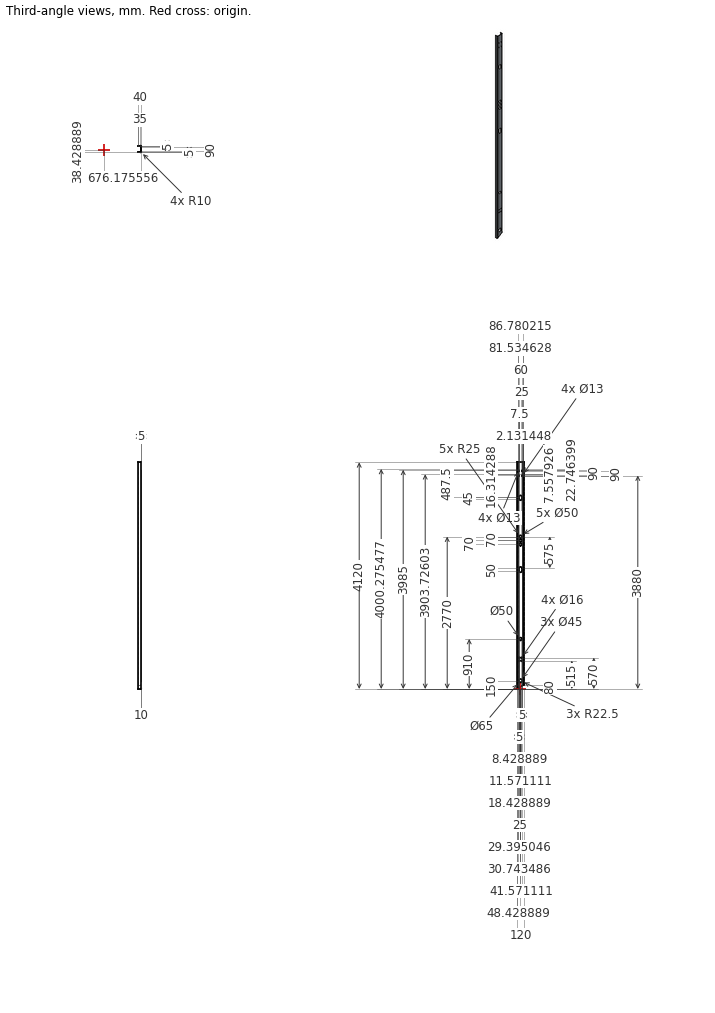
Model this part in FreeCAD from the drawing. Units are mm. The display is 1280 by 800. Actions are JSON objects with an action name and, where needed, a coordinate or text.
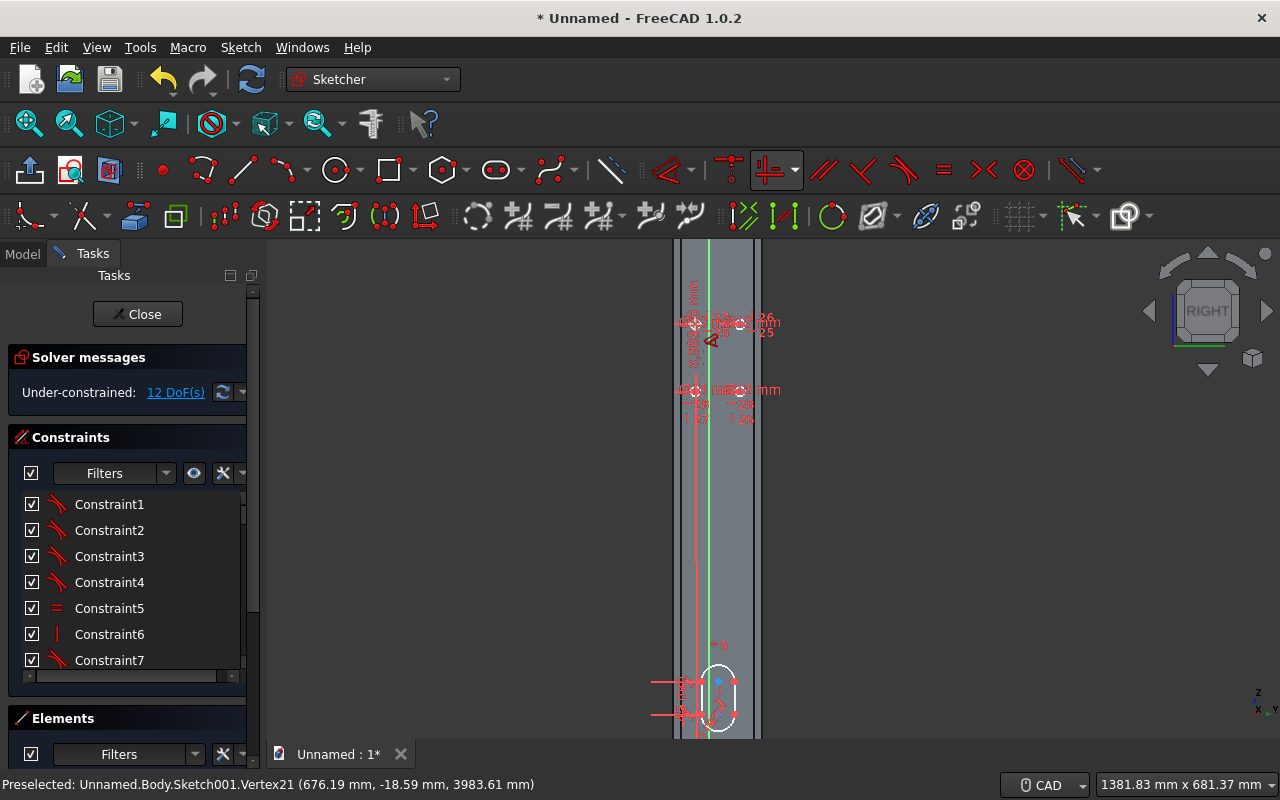
{"action": "left_click", "coordinate": [740, 324]}
{"action": "left_click", "coordinate": [728, 290]}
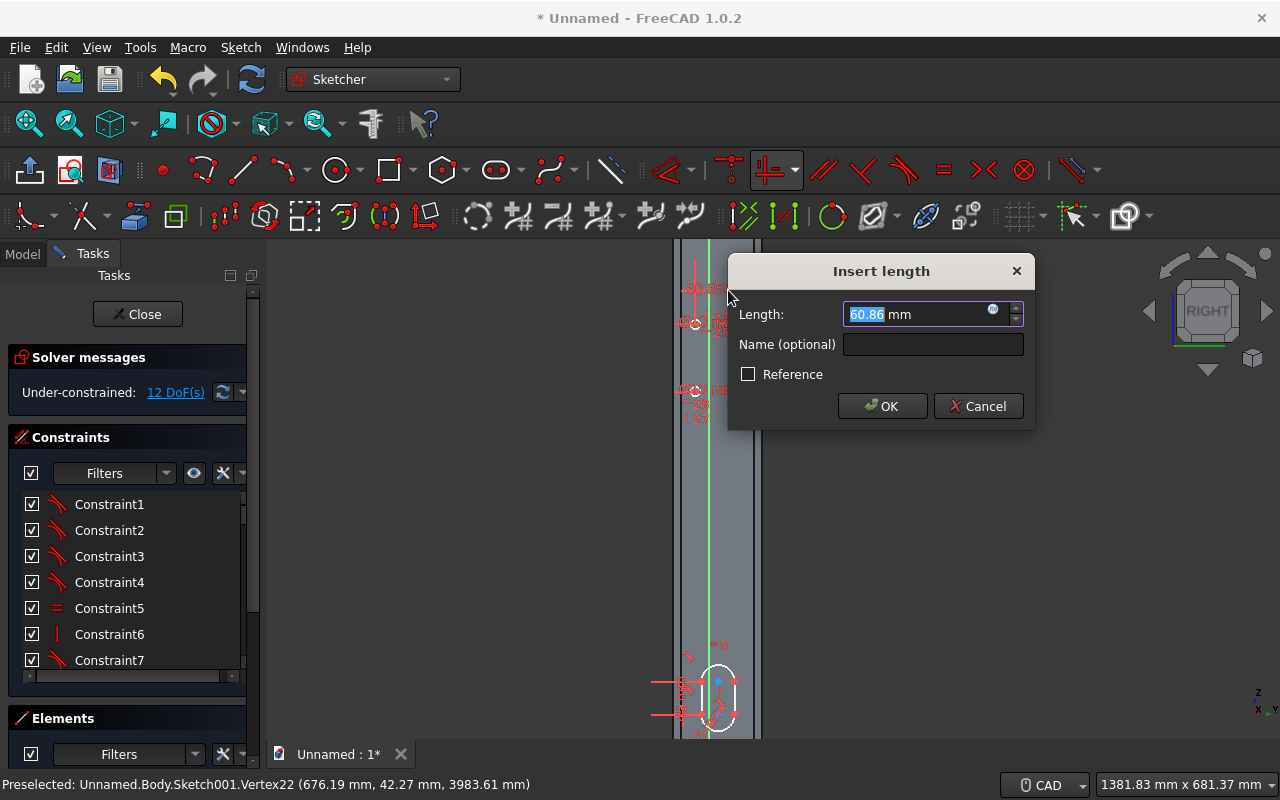
{"action": "type", "text": "60"}
{"action": "key", "text": "Return"}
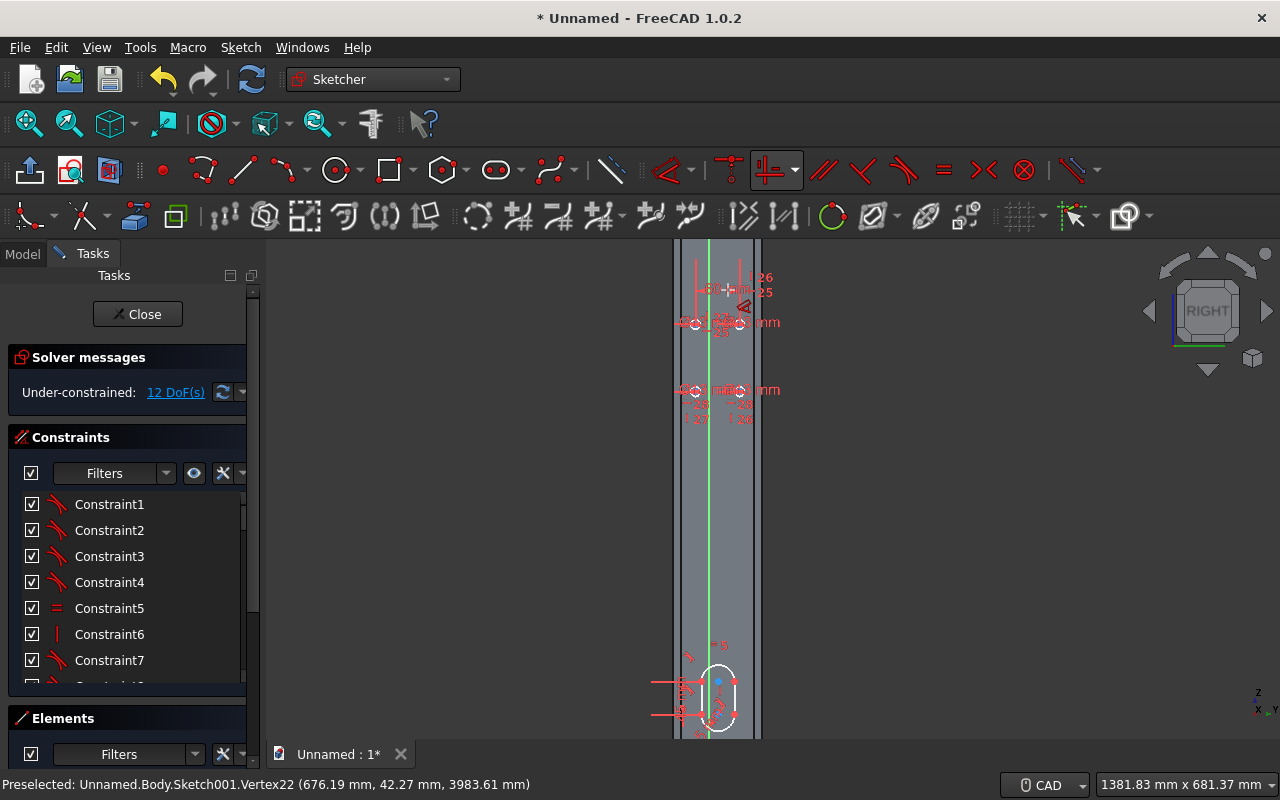
{"action": "left_click", "coordinate": [740, 324]}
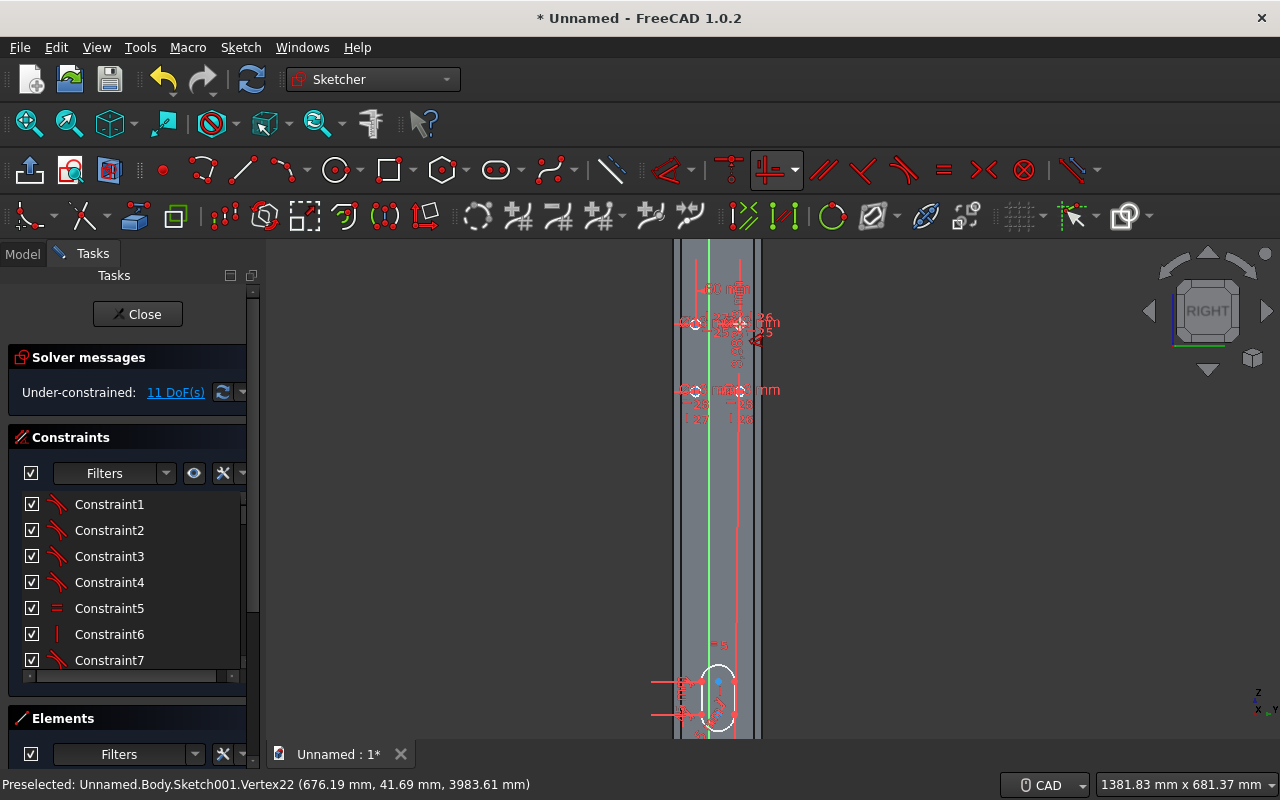
{"action": "left_click", "coordinate": [740, 392]}
{"action": "left_click", "coordinate": [774, 358]}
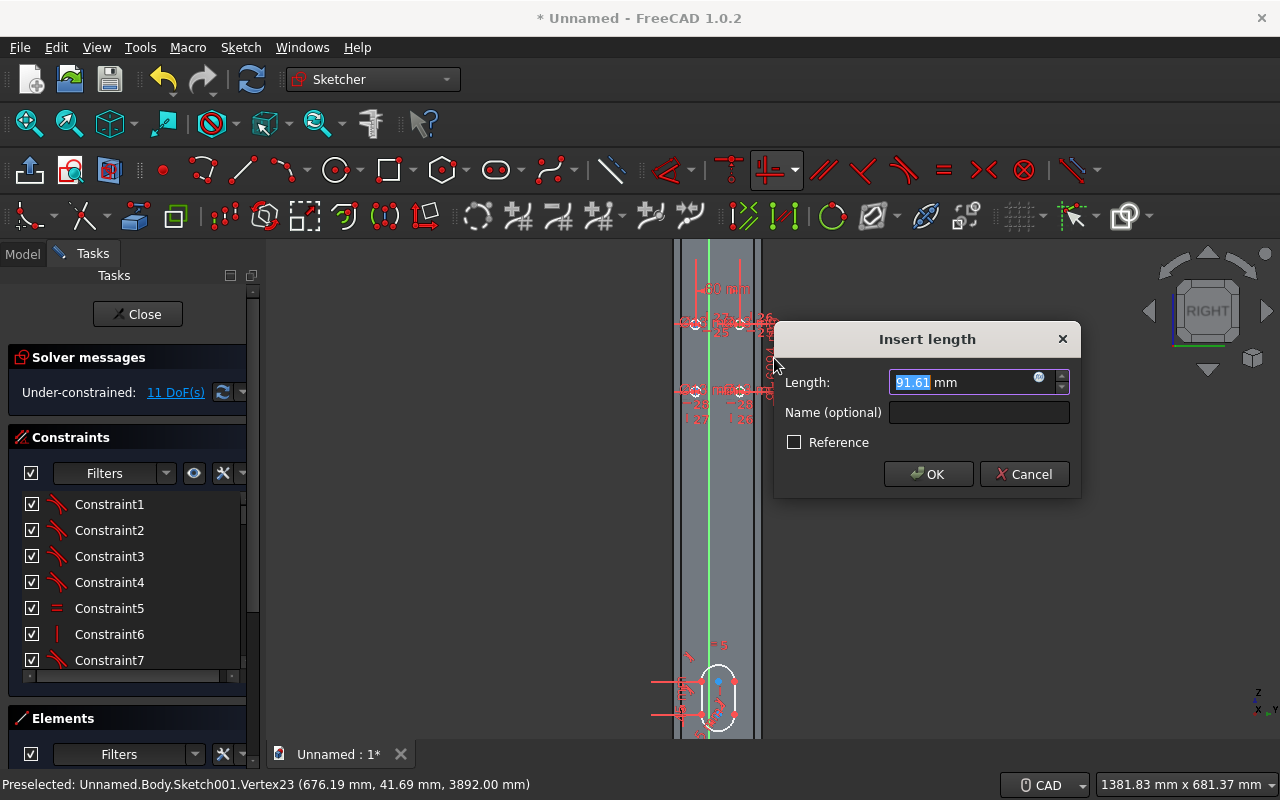
{"action": "type", "text": "90"}
{"action": "key", "text": "Return"}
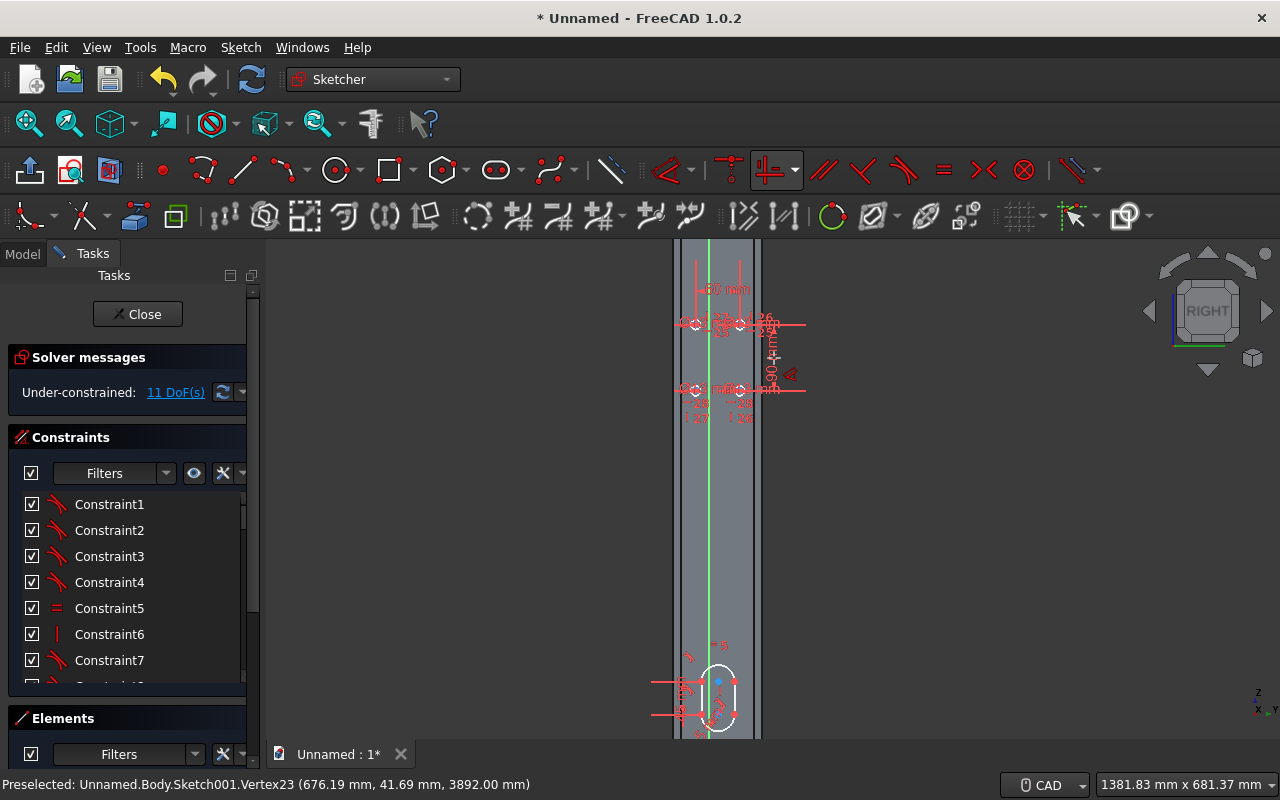
{"action": "scroll", "coordinate": [703, 328], "scroll_direction": "down", "scroll_amount": 11}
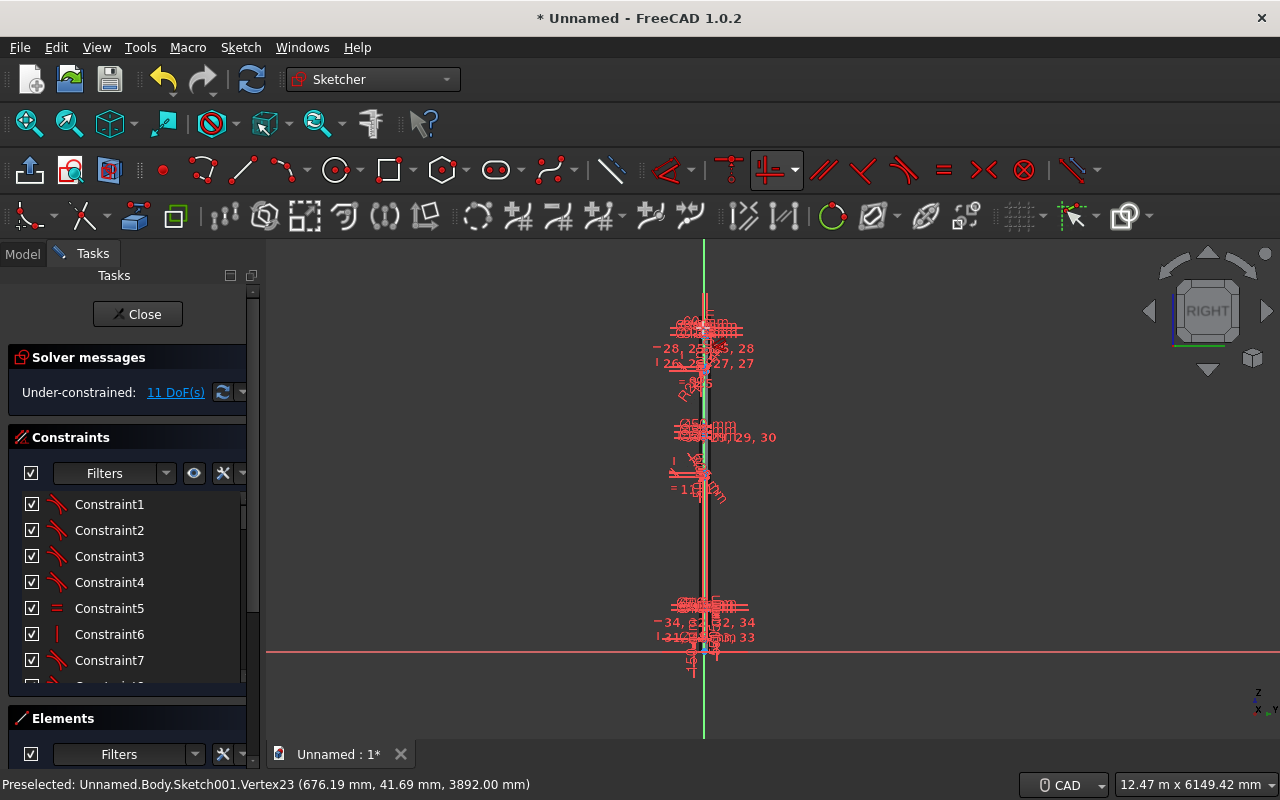
{"action": "scroll", "coordinate": [707, 473], "scroll_direction": "up", "scroll_amount": 15}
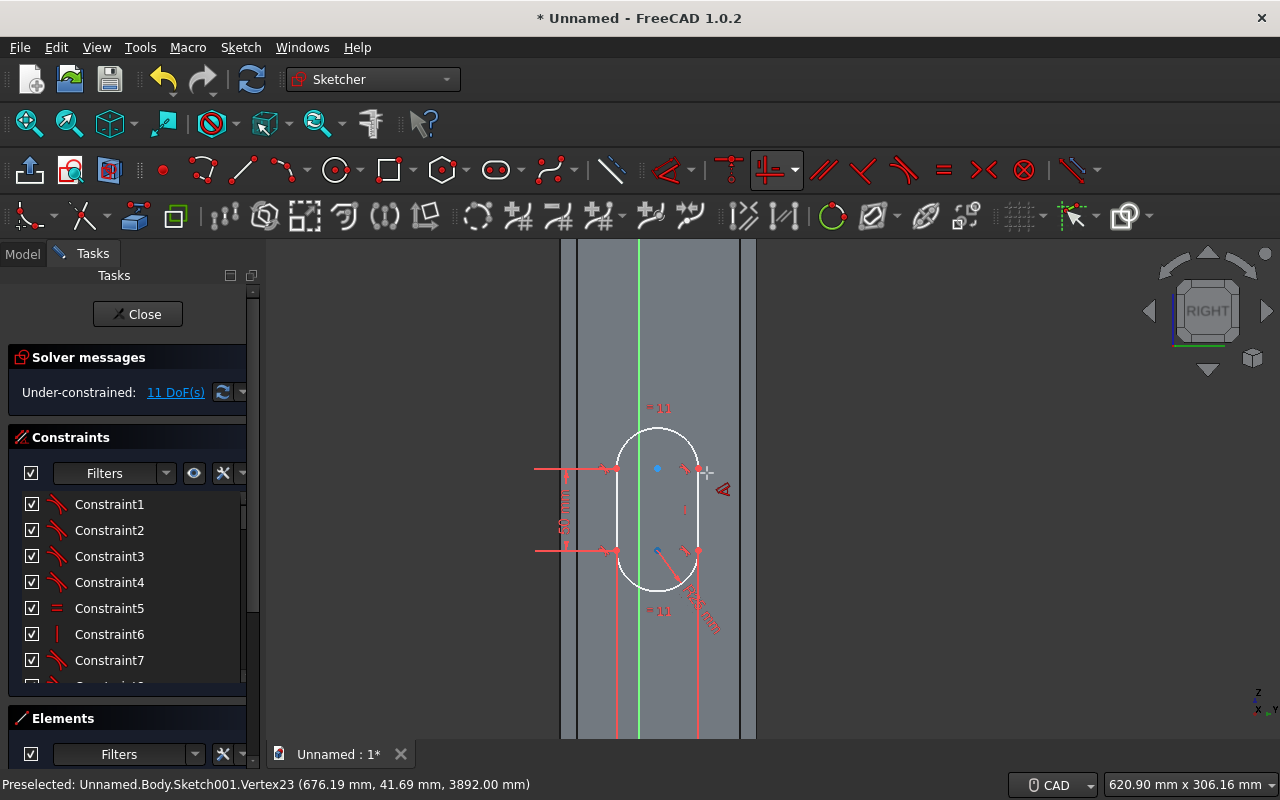
{"action": "left_click", "coordinate": [698, 469]}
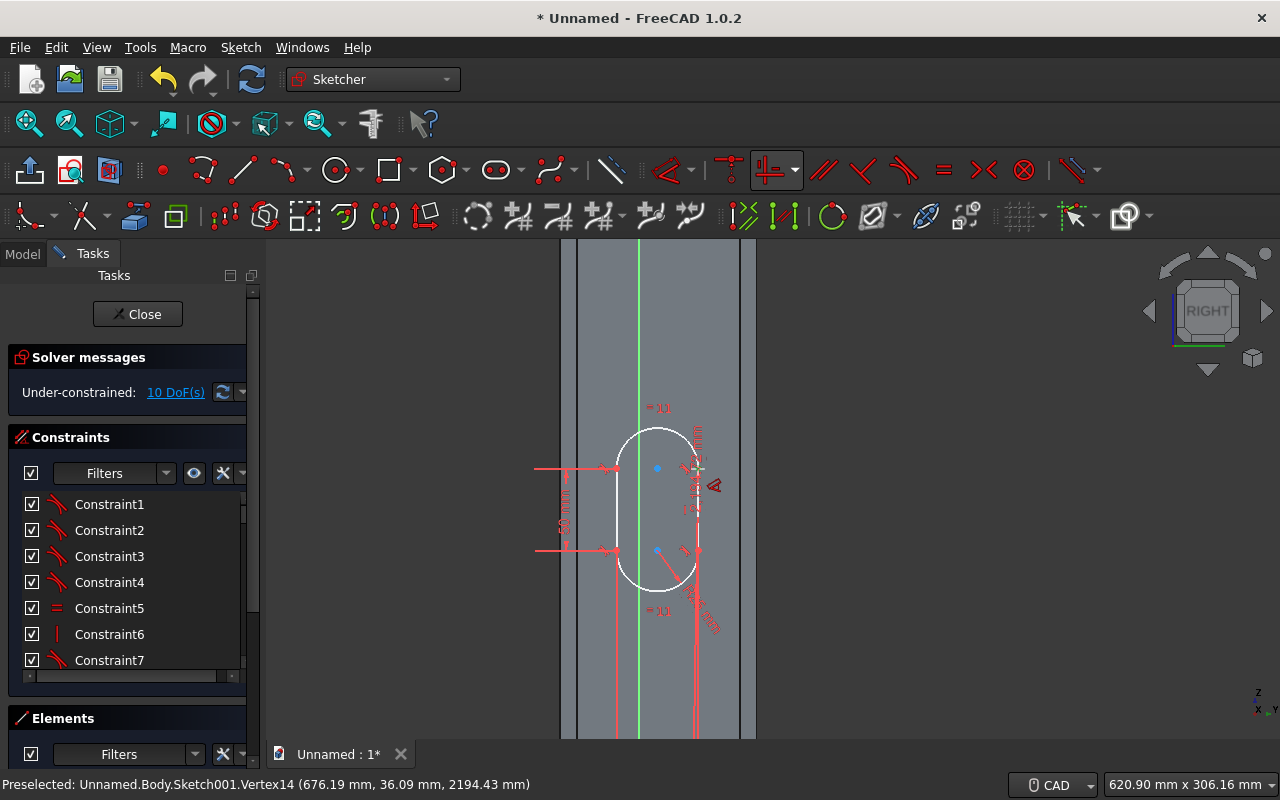
{"action": "scroll", "coordinate": [707, 473], "scroll_direction": "down", "scroll_amount": 15}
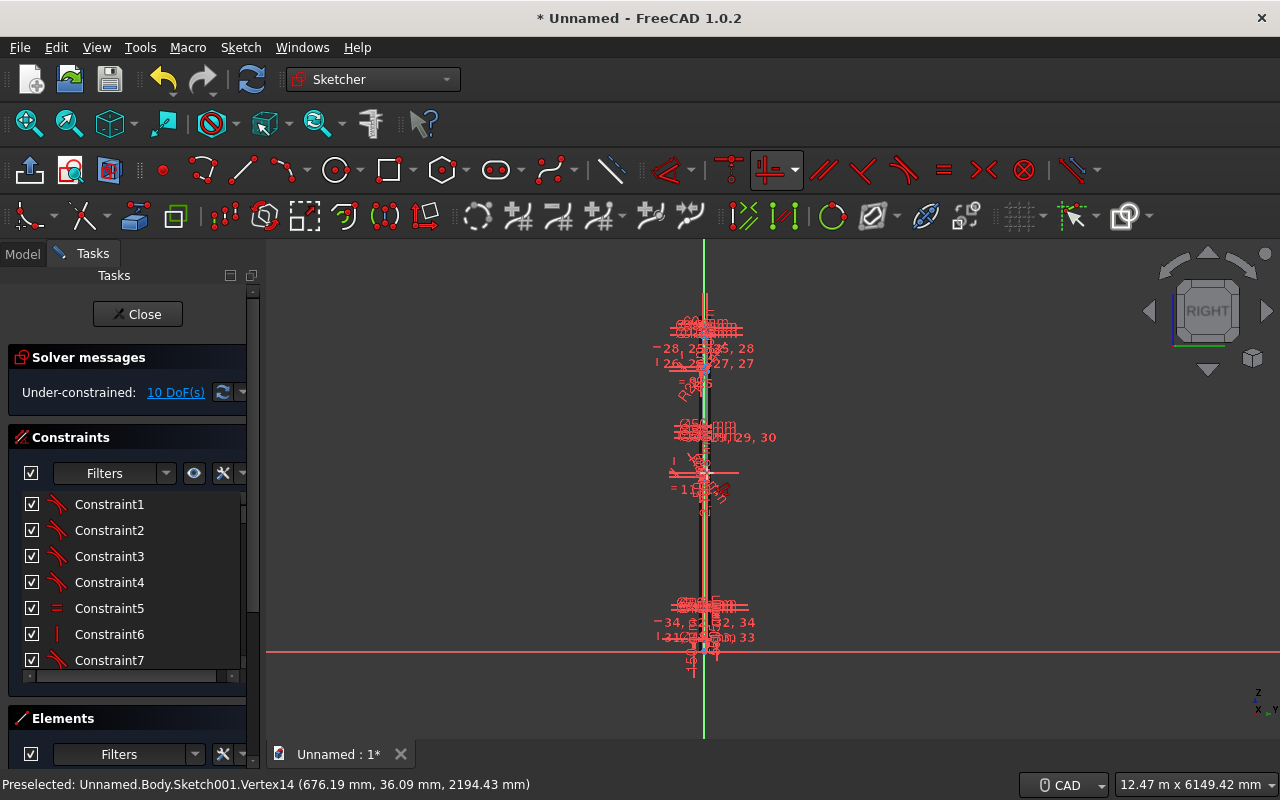
{"action": "scroll", "coordinate": [705, 426], "scroll_direction": "up", "scroll_amount": 15}